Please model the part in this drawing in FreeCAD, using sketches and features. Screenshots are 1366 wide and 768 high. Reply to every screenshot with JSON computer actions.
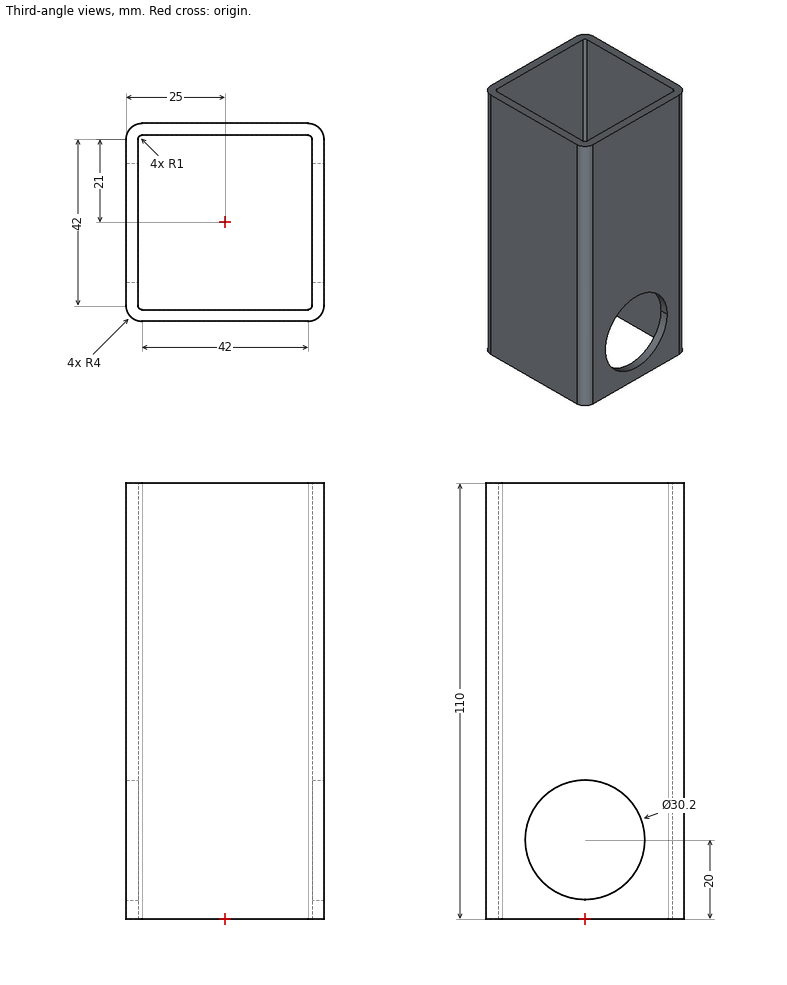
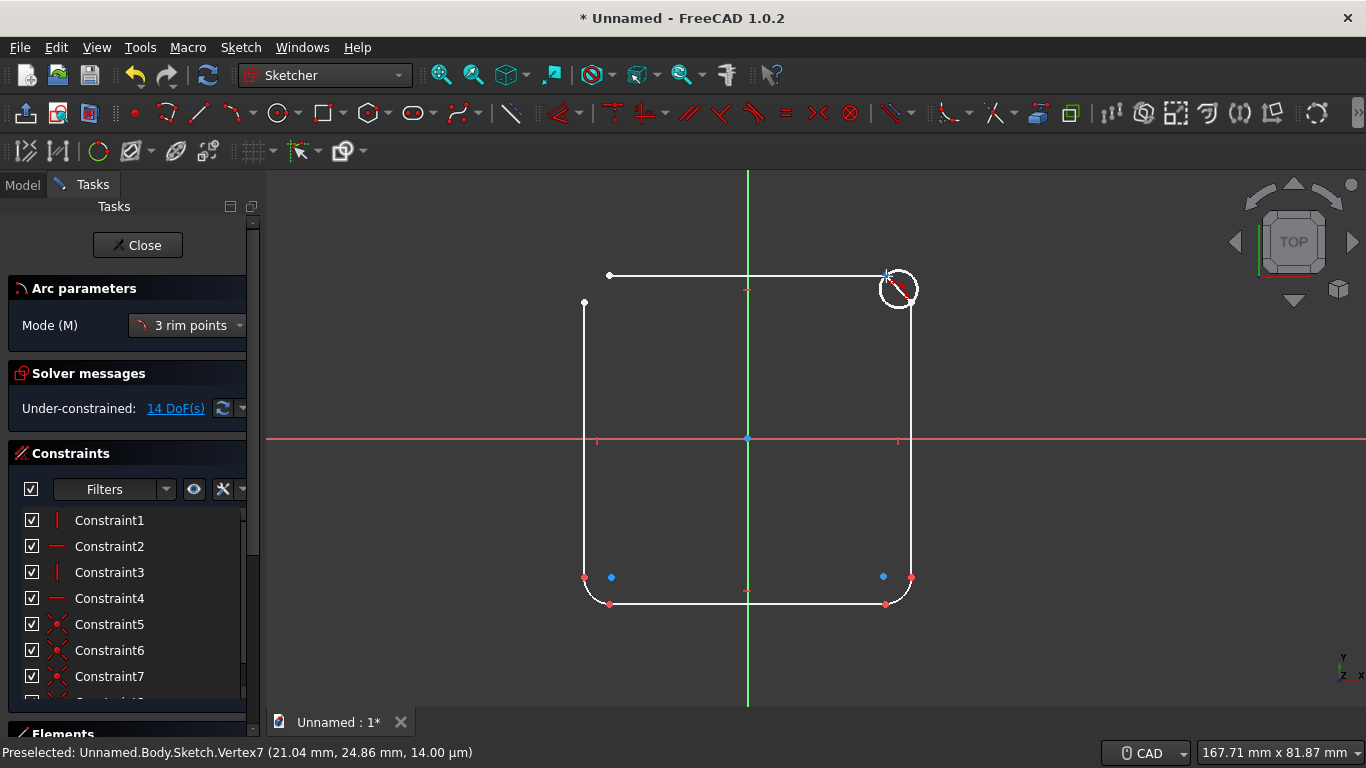
{"action": "scroll", "coordinate": [904, 283], "scroll_direction": "up", "scroll_amount": 4}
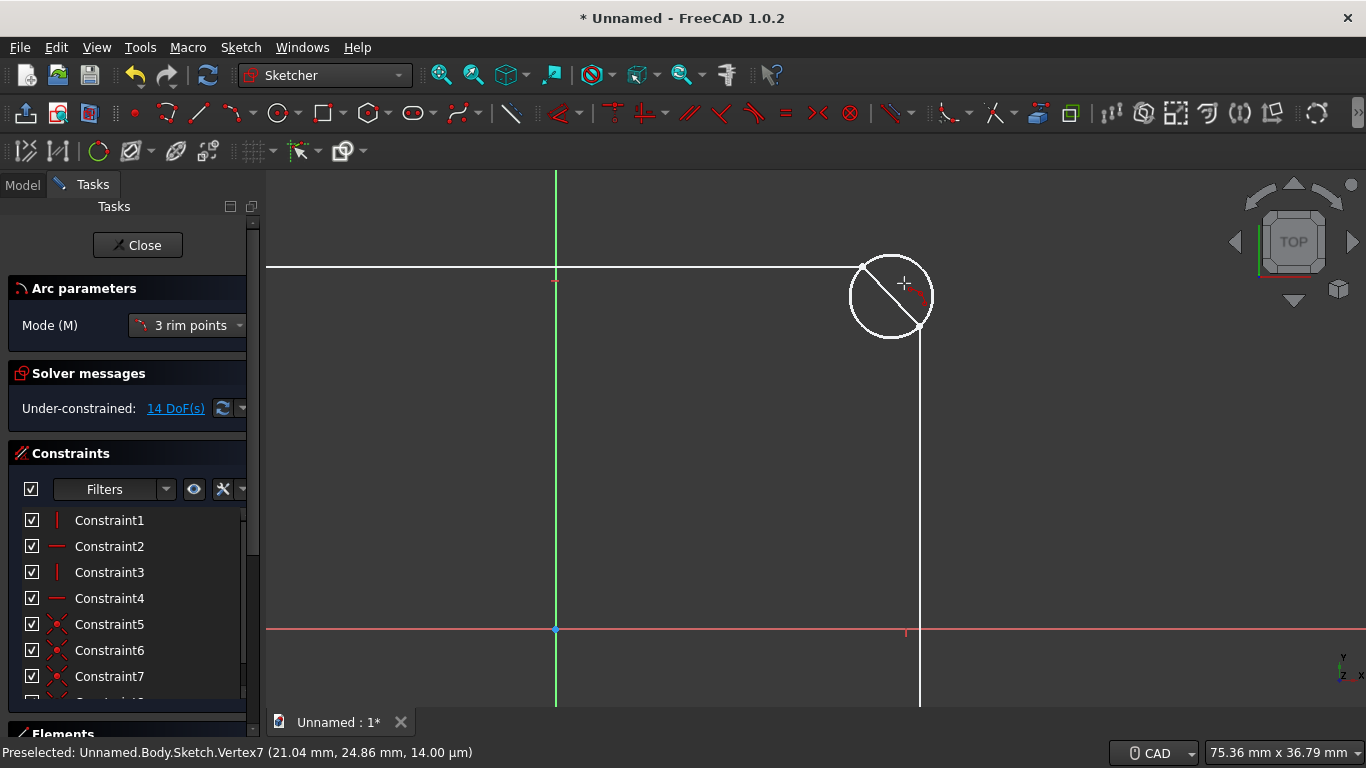
{"action": "left_click", "coordinate": [903, 282]}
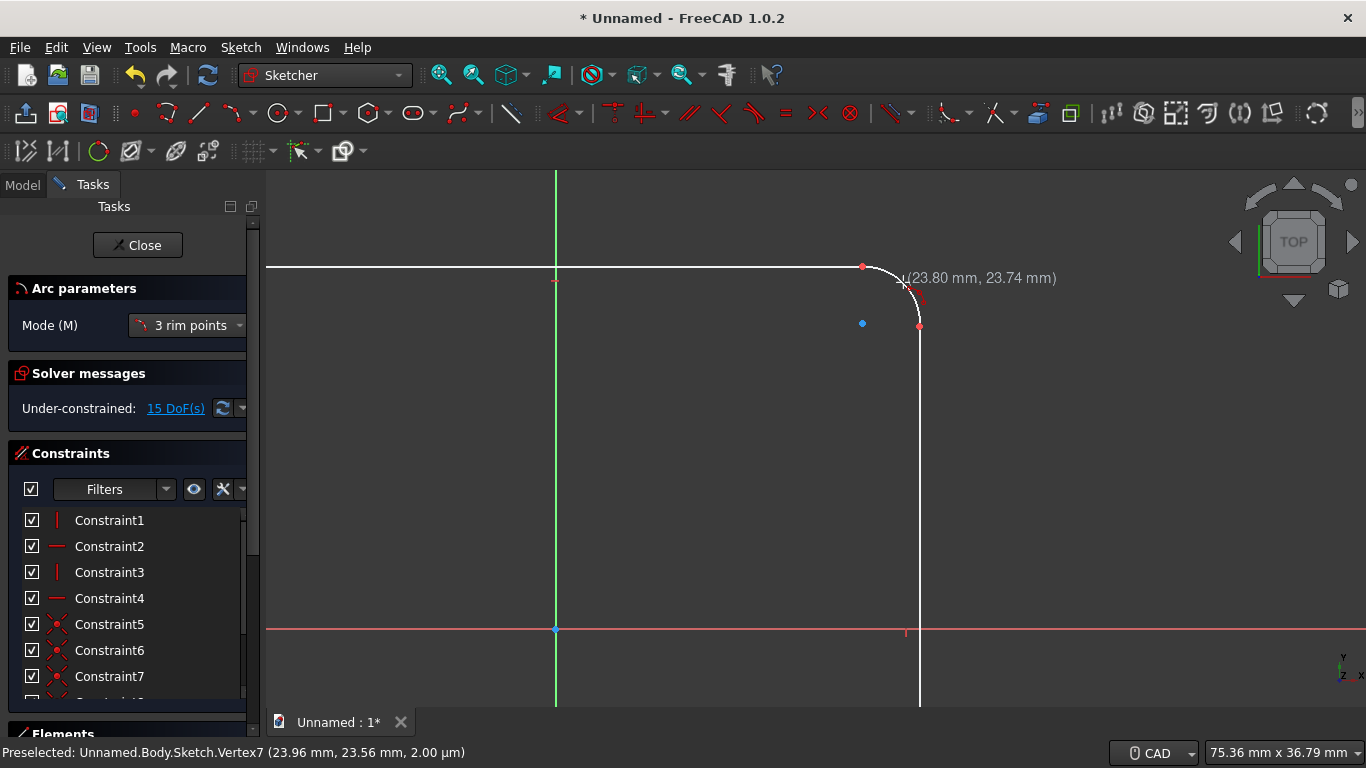
{"action": "scroll", "coordinate": [904, 283], "scroll_direction": "down", "scroll_amount": 4}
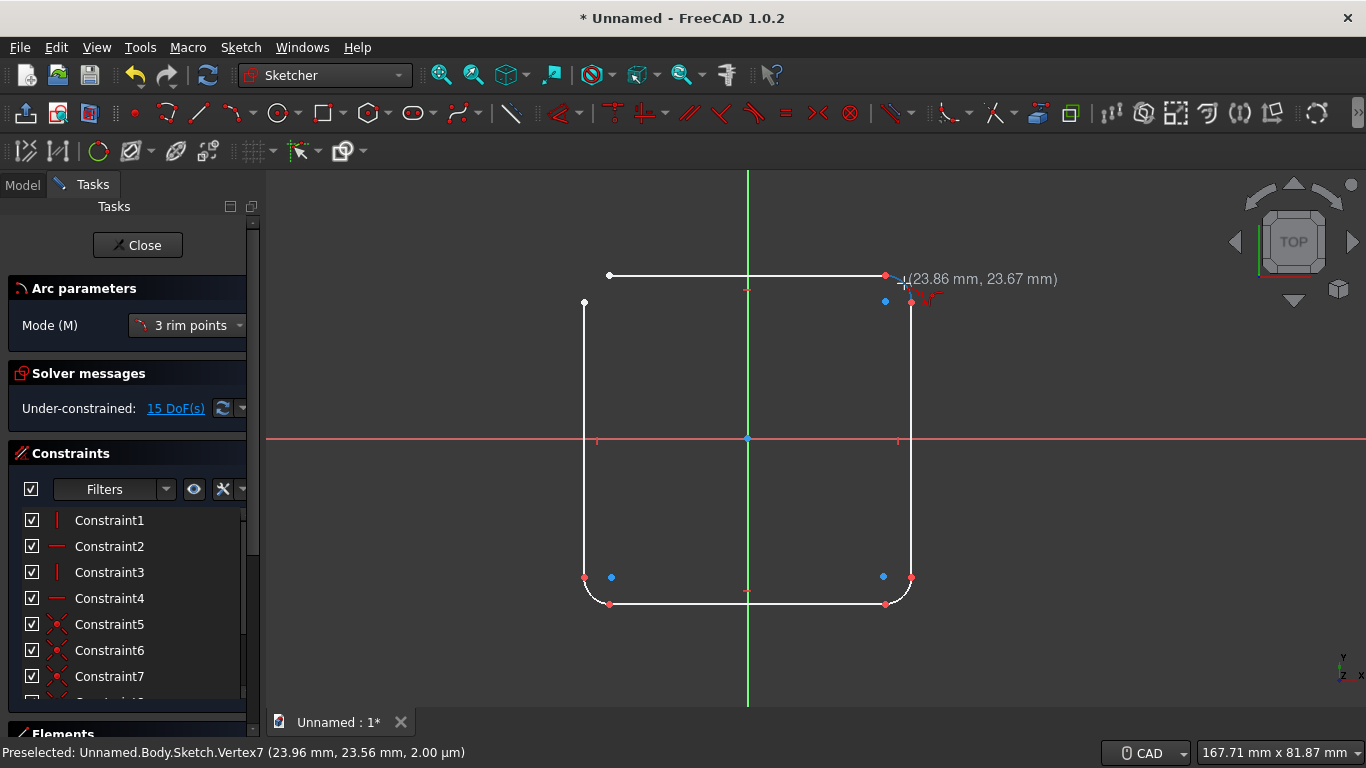
{"action": "left_click", "coordinate": [610, 276]}
{"action": "left_click", "coordinate": [584, 303]}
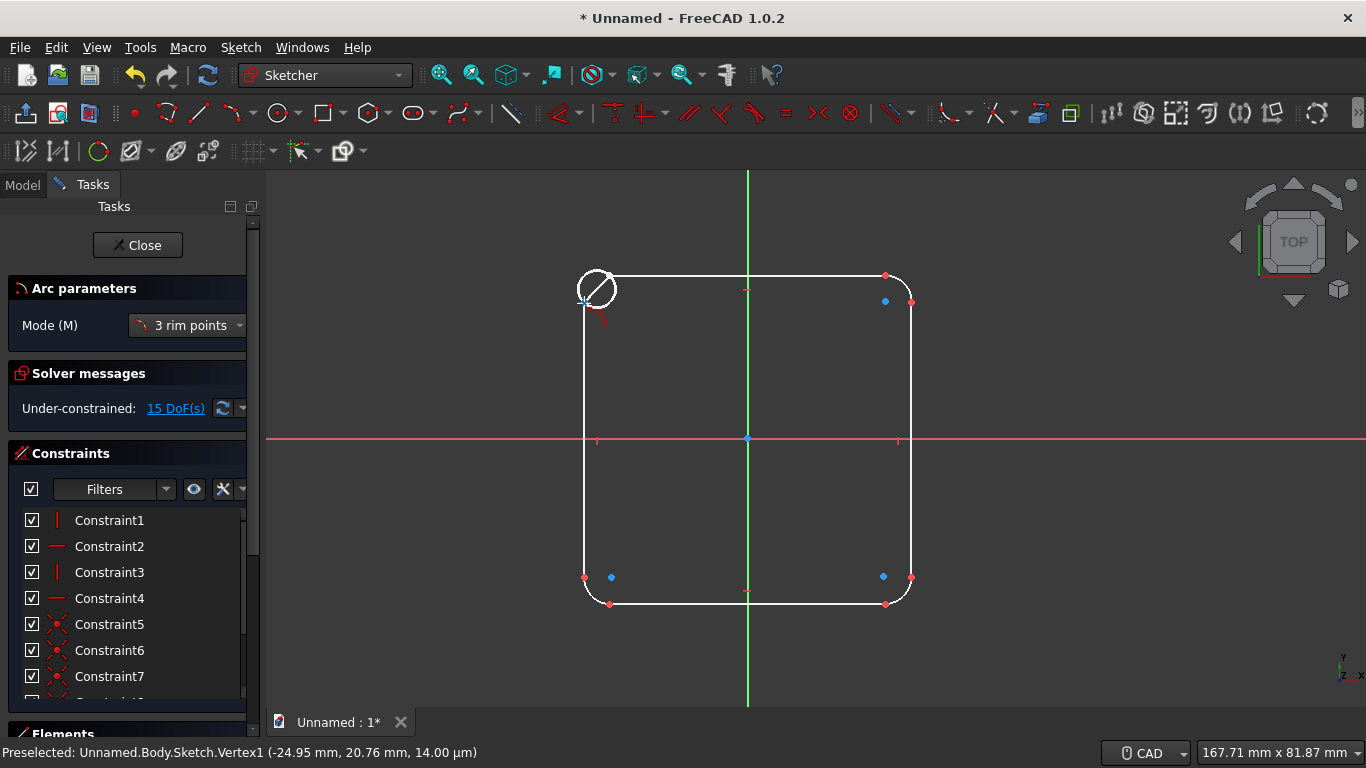
{"action": "scroll", "coordinate": [592, 283], "scroll_direction": "up", "scroll_amount": 4}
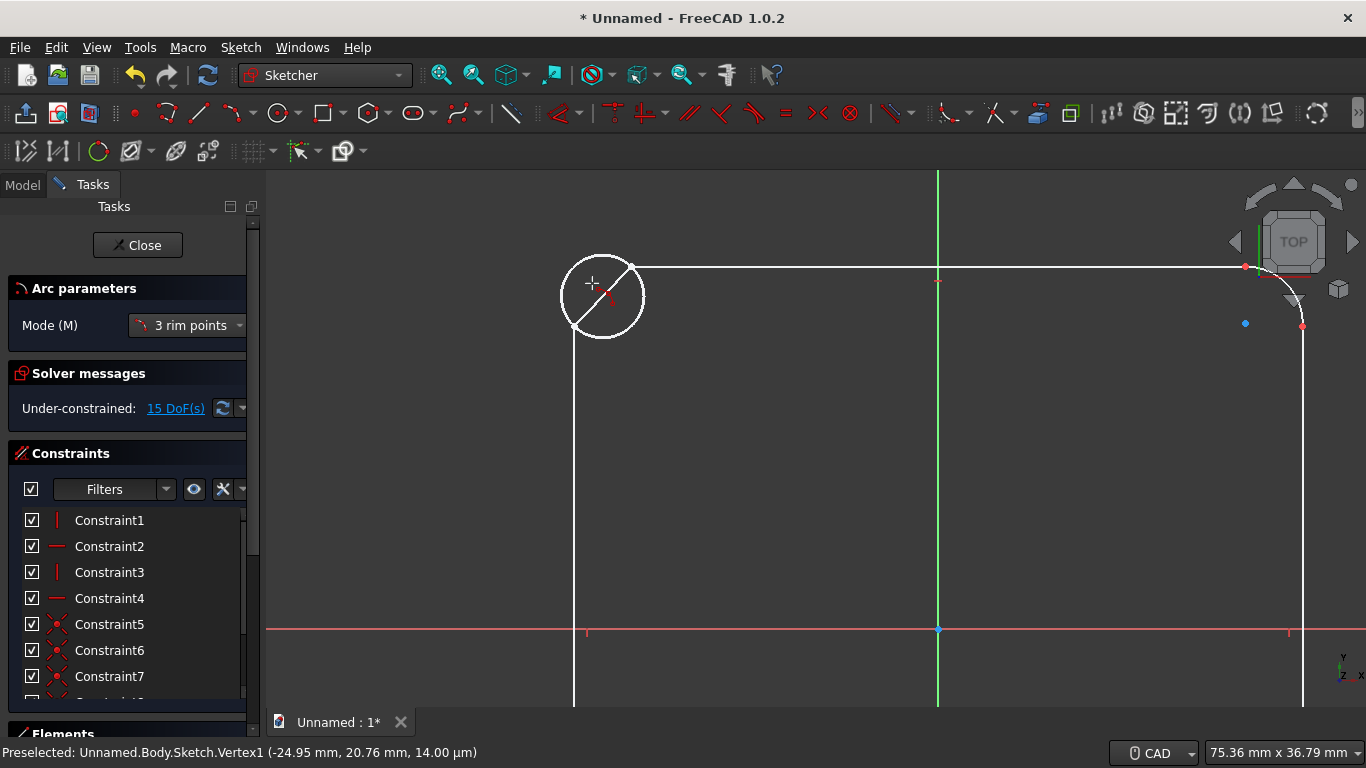
{"action": "left_click", "coordinate": [591, 282]}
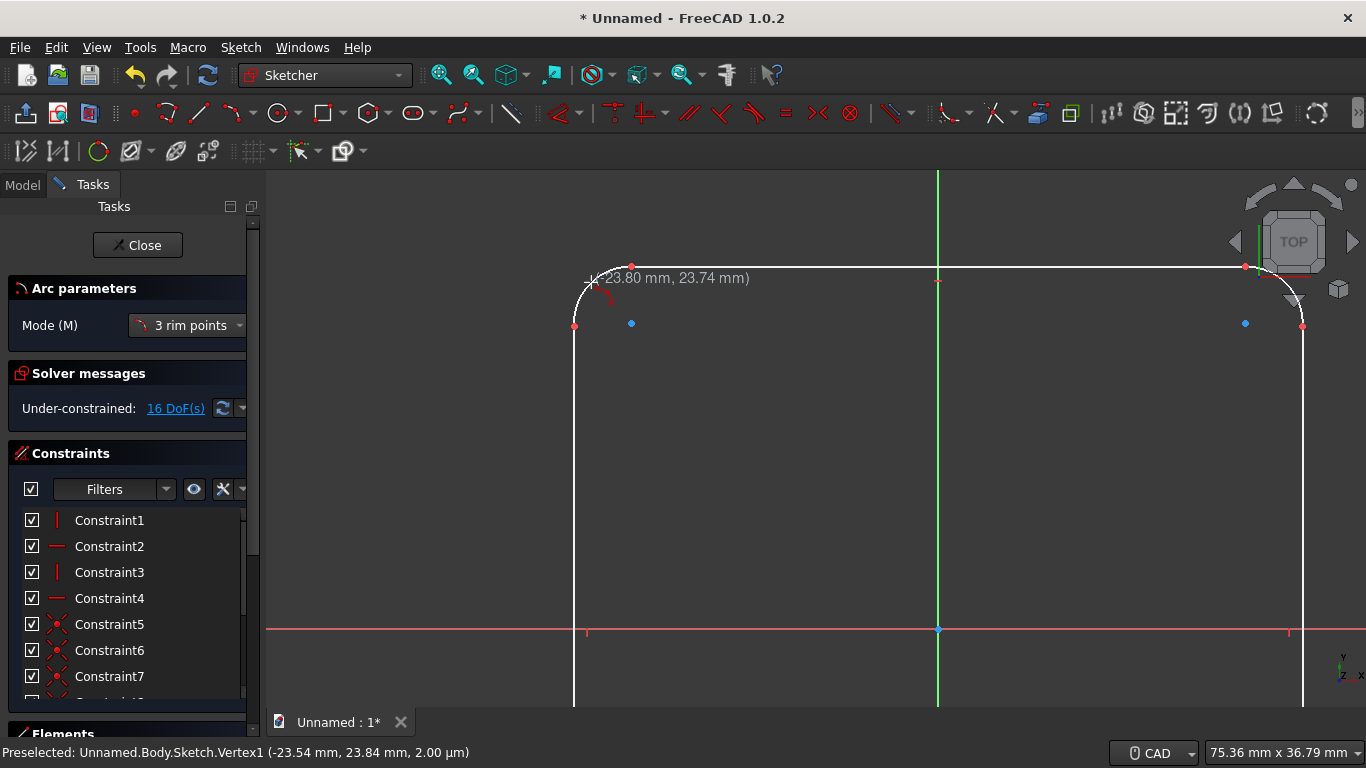
{"action": "left_click", "coordinate": [200, 114]}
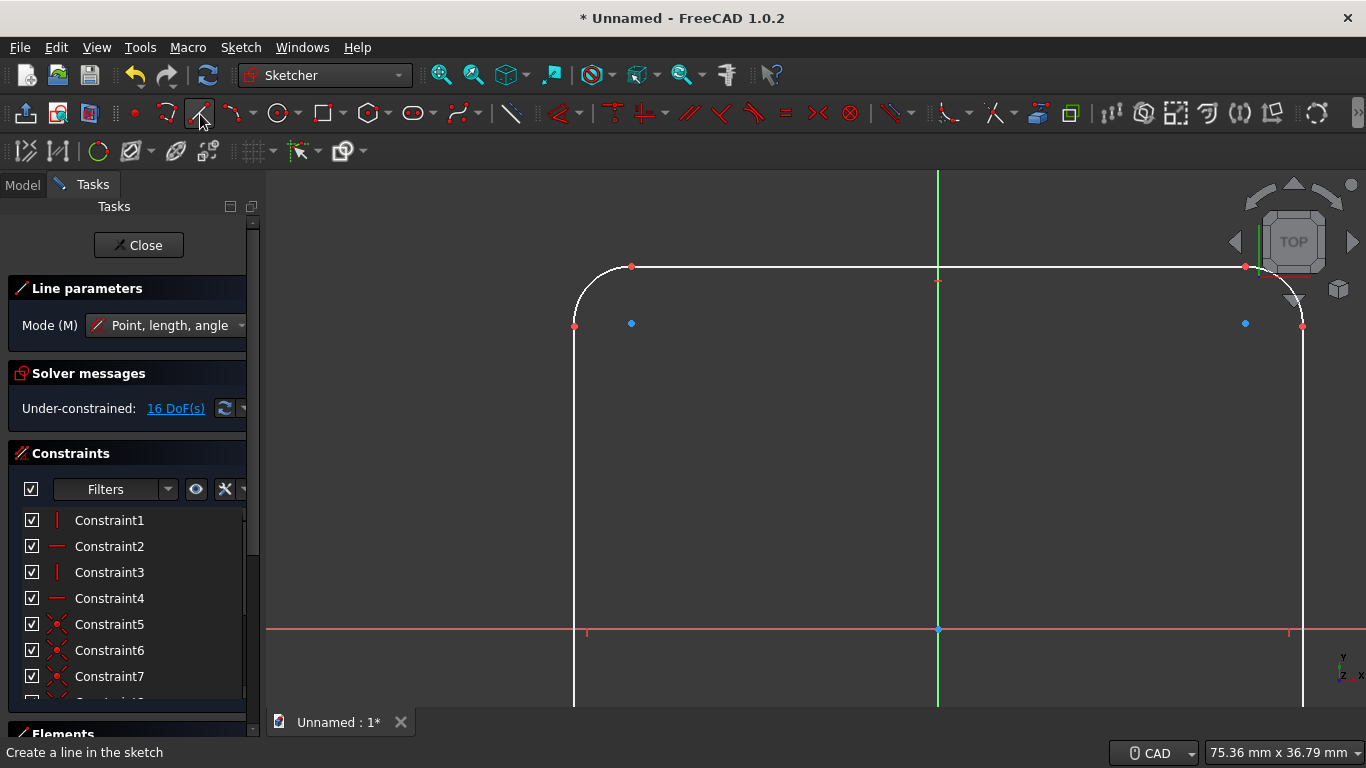
{"action": "scroll", "coordinate": [592, 283], "scroll_direction": "down", "scroll_amount": 4}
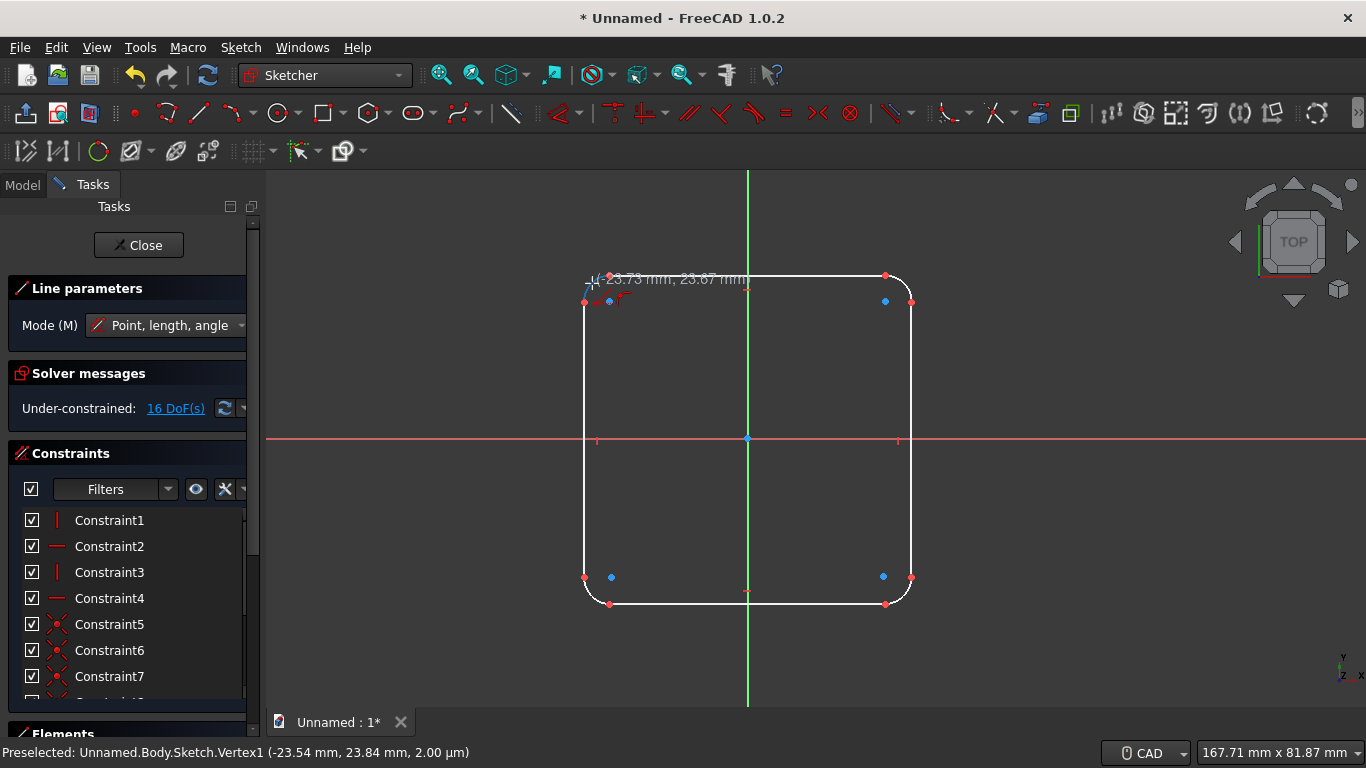
{"action": "scroll", "coordinate": [604, 577], "scroll_direction": "up", "scroll_amount": 5}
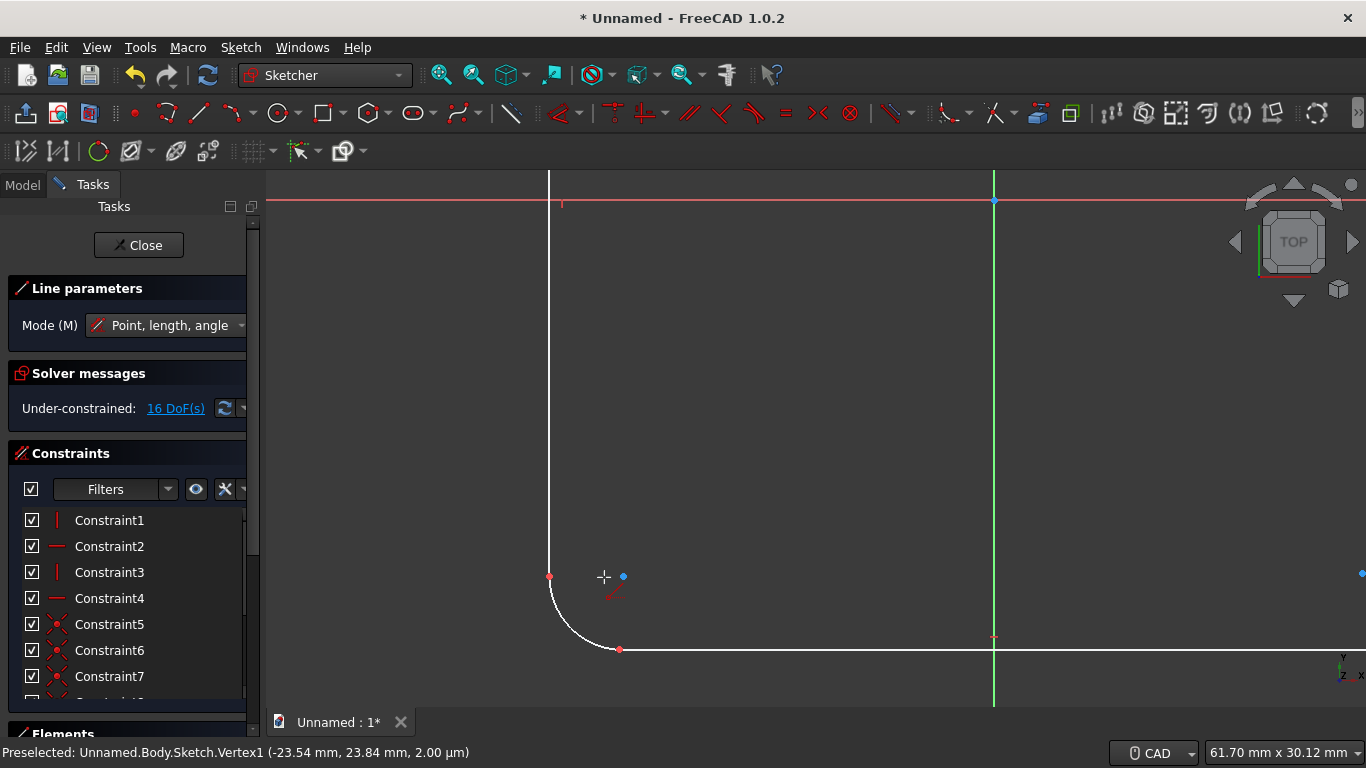
{"action": "left_click", "coordinate": [602, 574]}